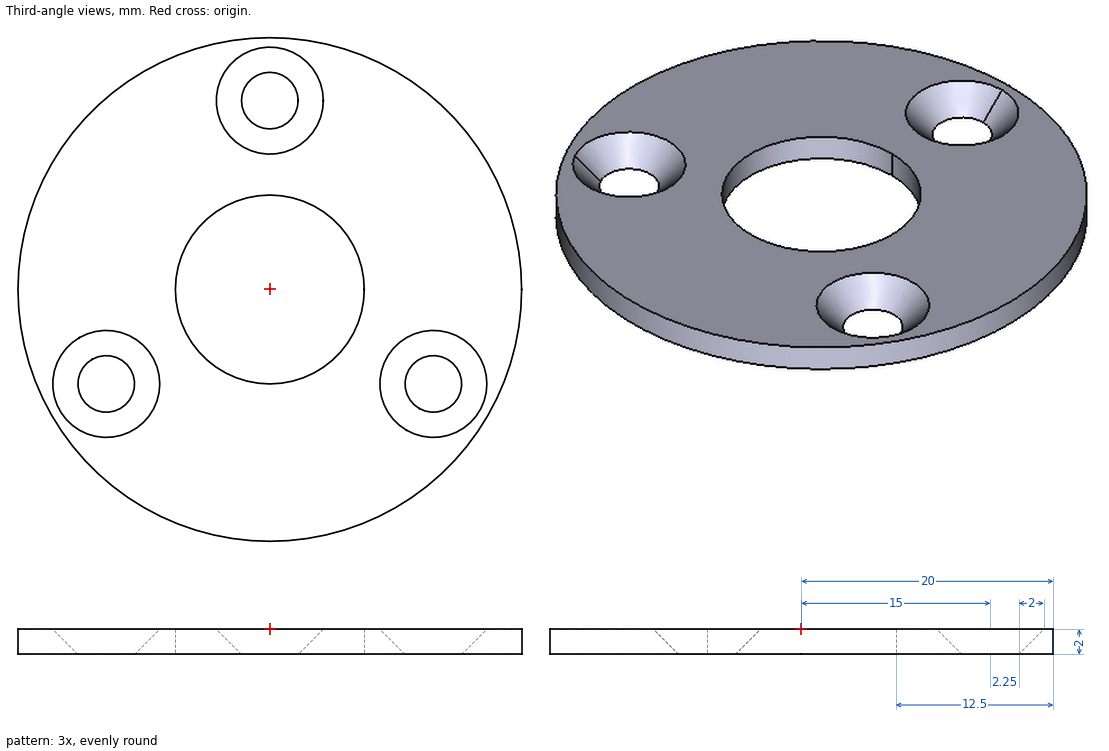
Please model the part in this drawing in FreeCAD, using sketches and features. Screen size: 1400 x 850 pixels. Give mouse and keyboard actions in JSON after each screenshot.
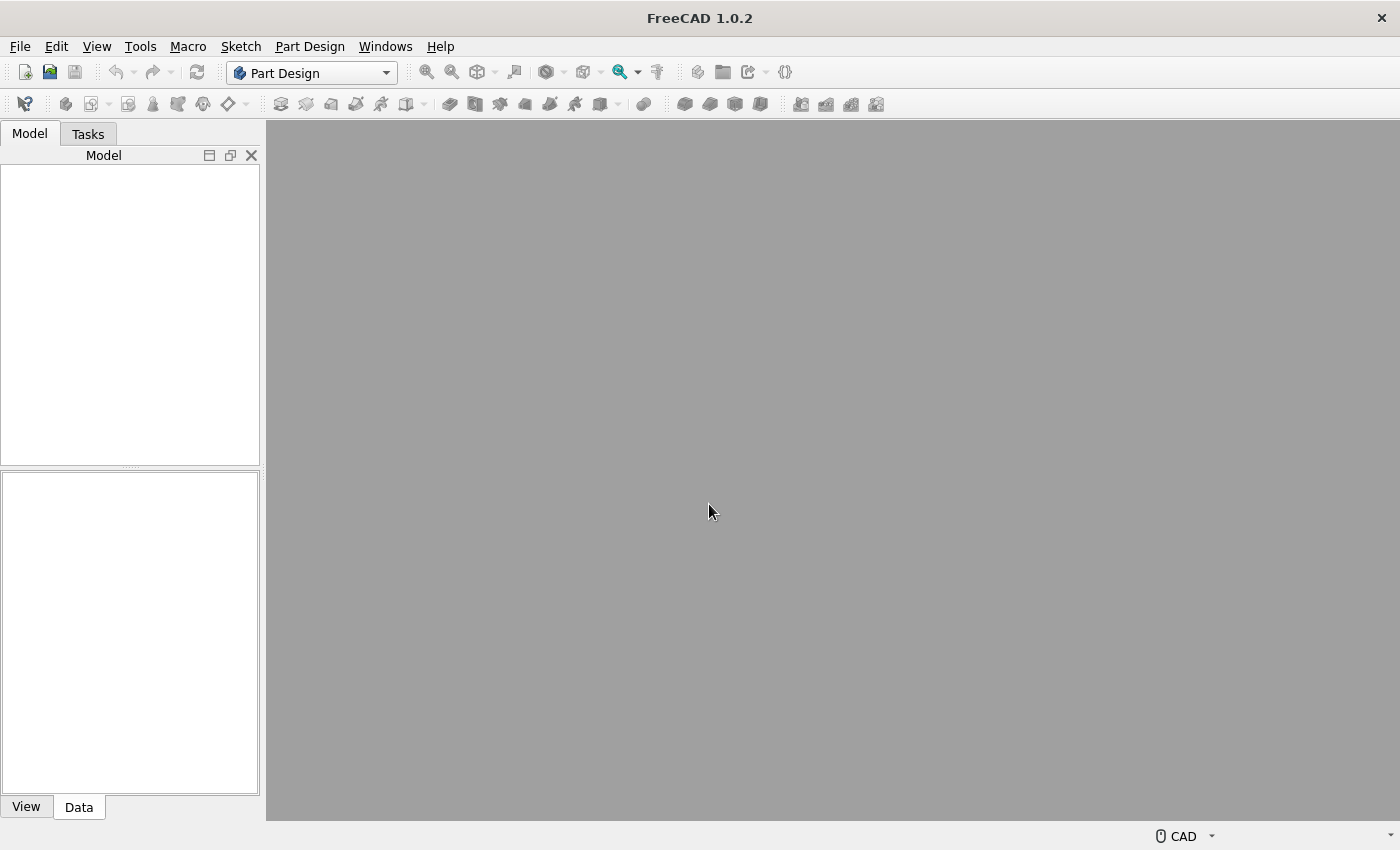
{"action": "left_click", "coordinate": [25, 72]}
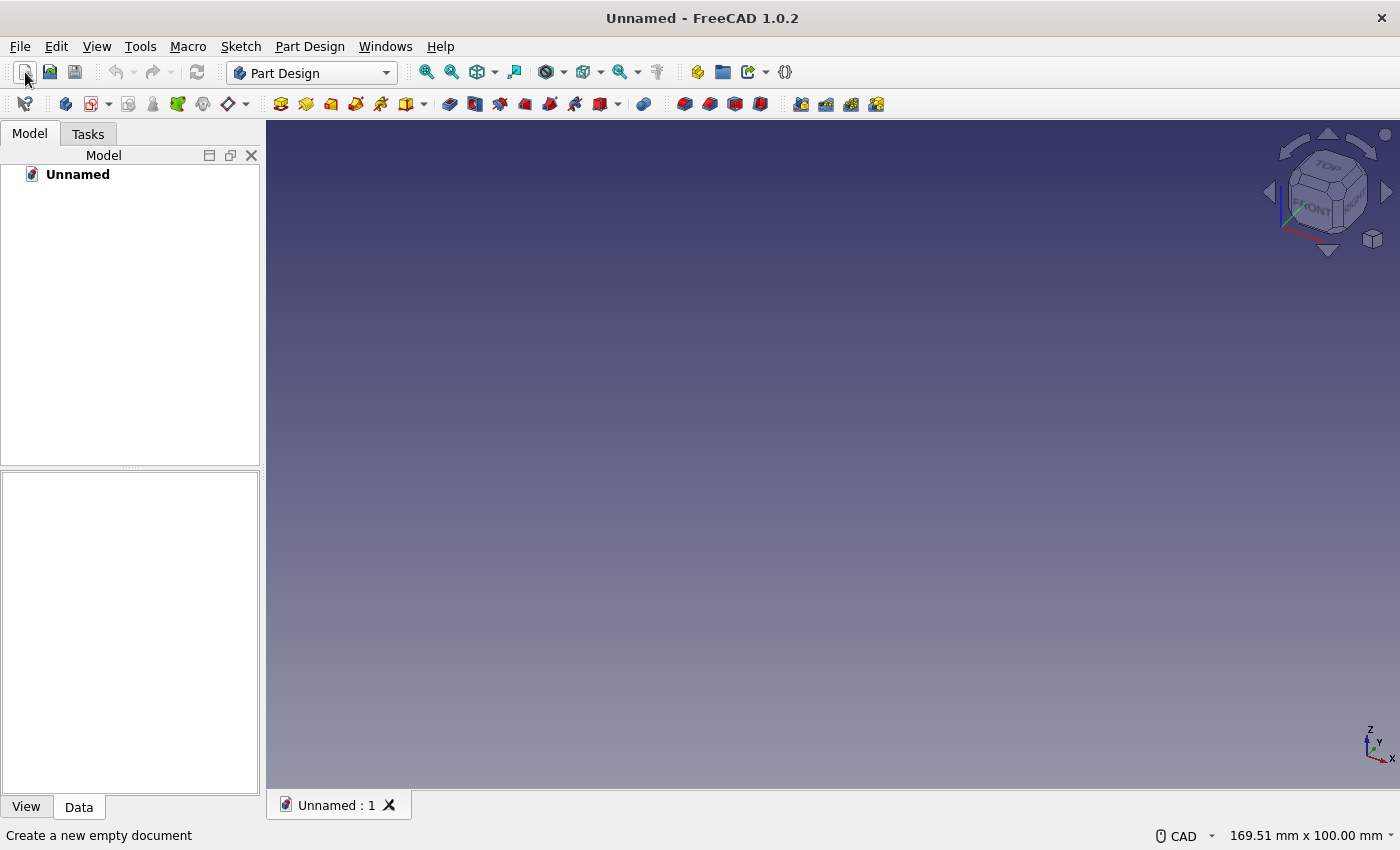
{"action": "left_click", "coordinate": [90, 104]}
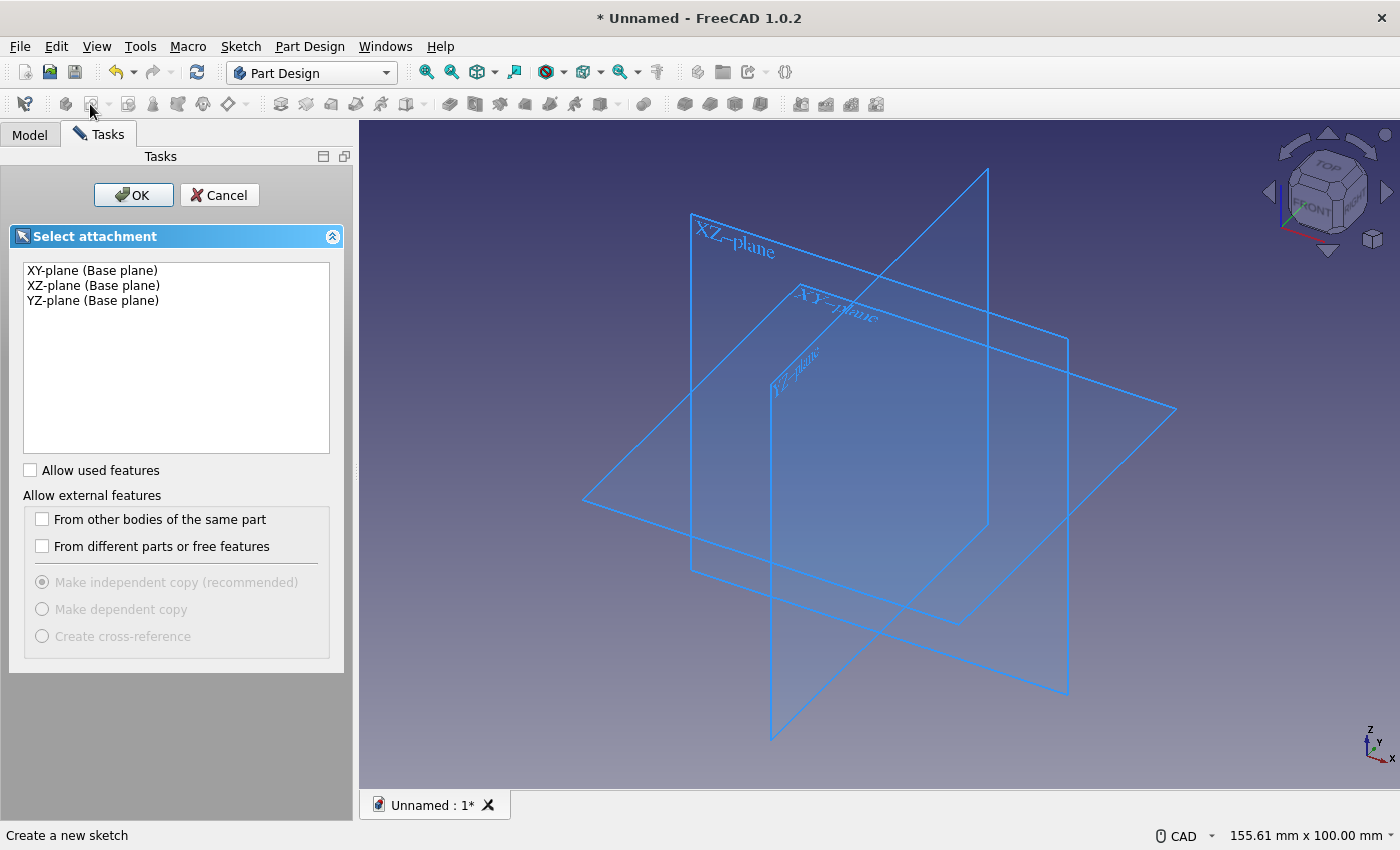
{"action": "left_click", "coordinate": [84, 300]}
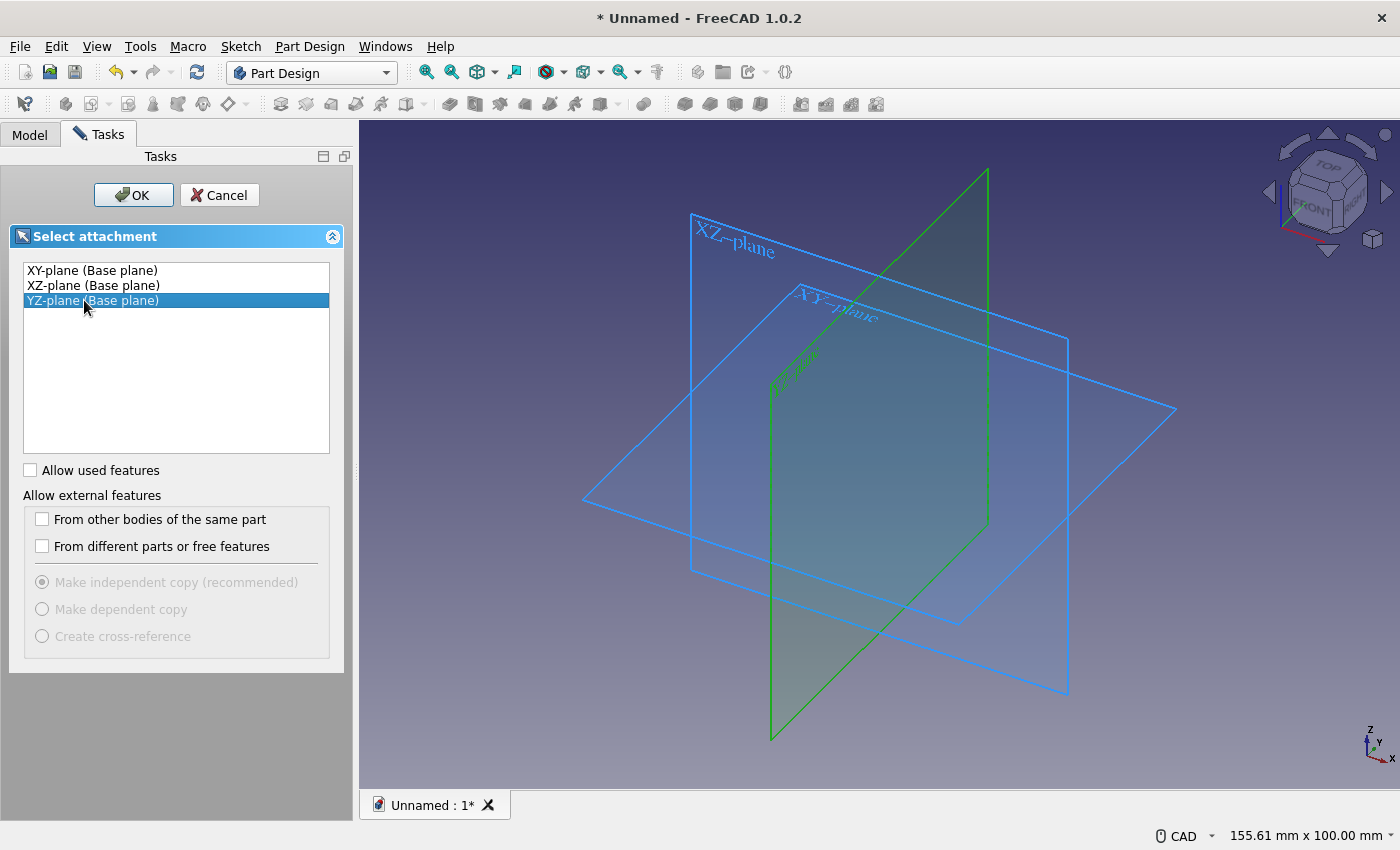
{"action": "left_click", "coordinate": [134, 195]}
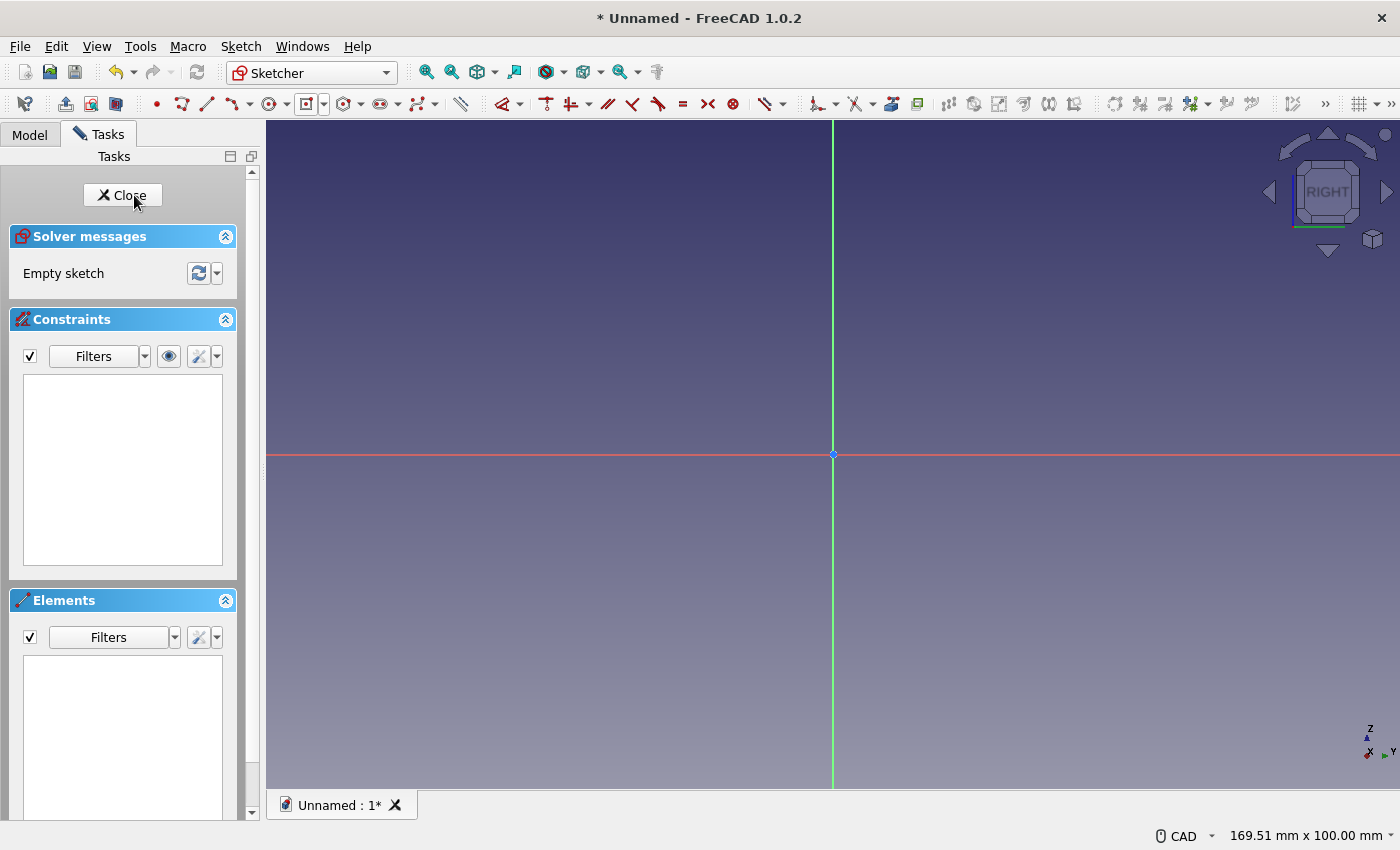
{"action": "scroll", "coordinate": [934, 463], "scroll_direction": "up", "scroll_amount": 8}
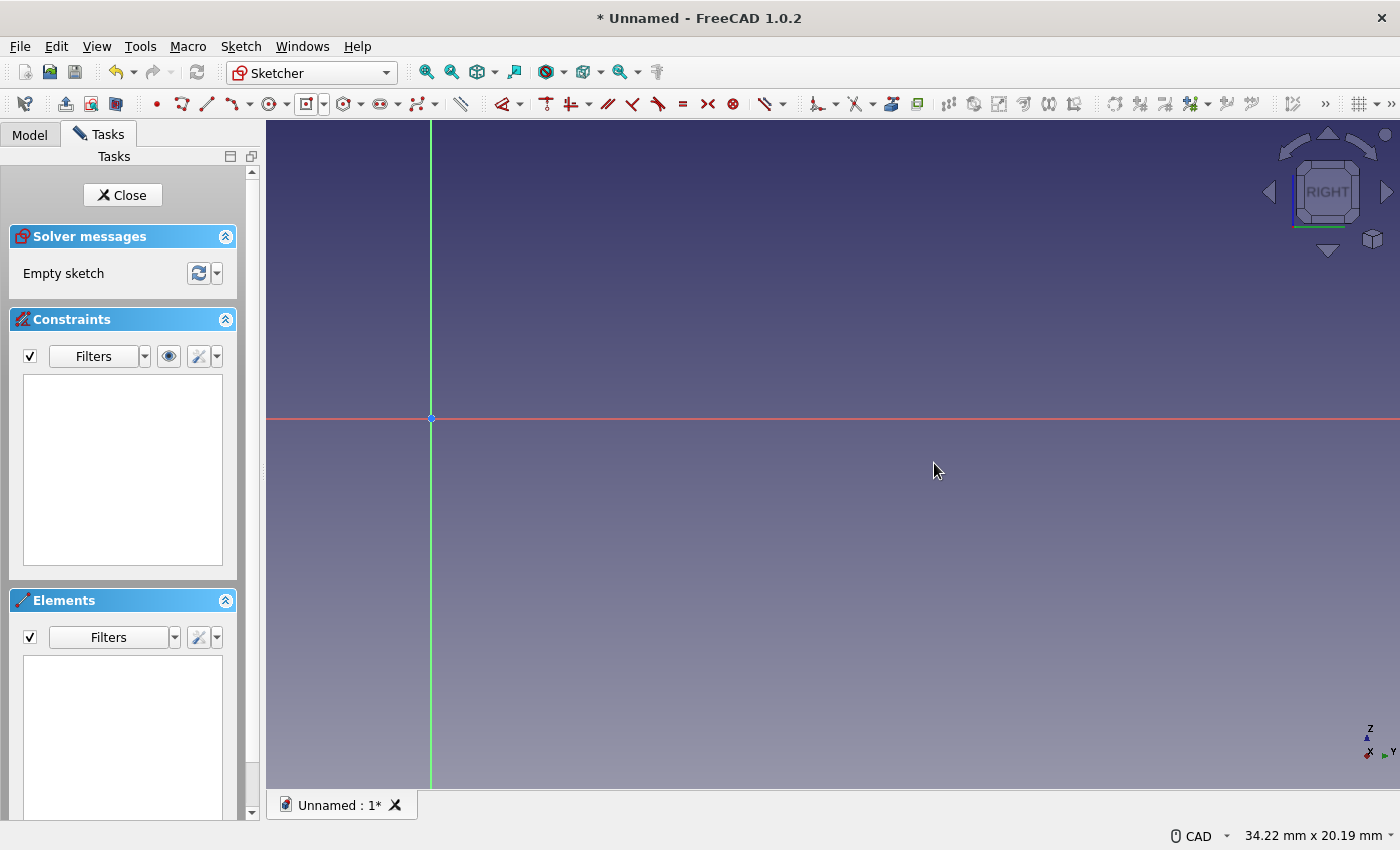
{"action": "key", "text": "g r"}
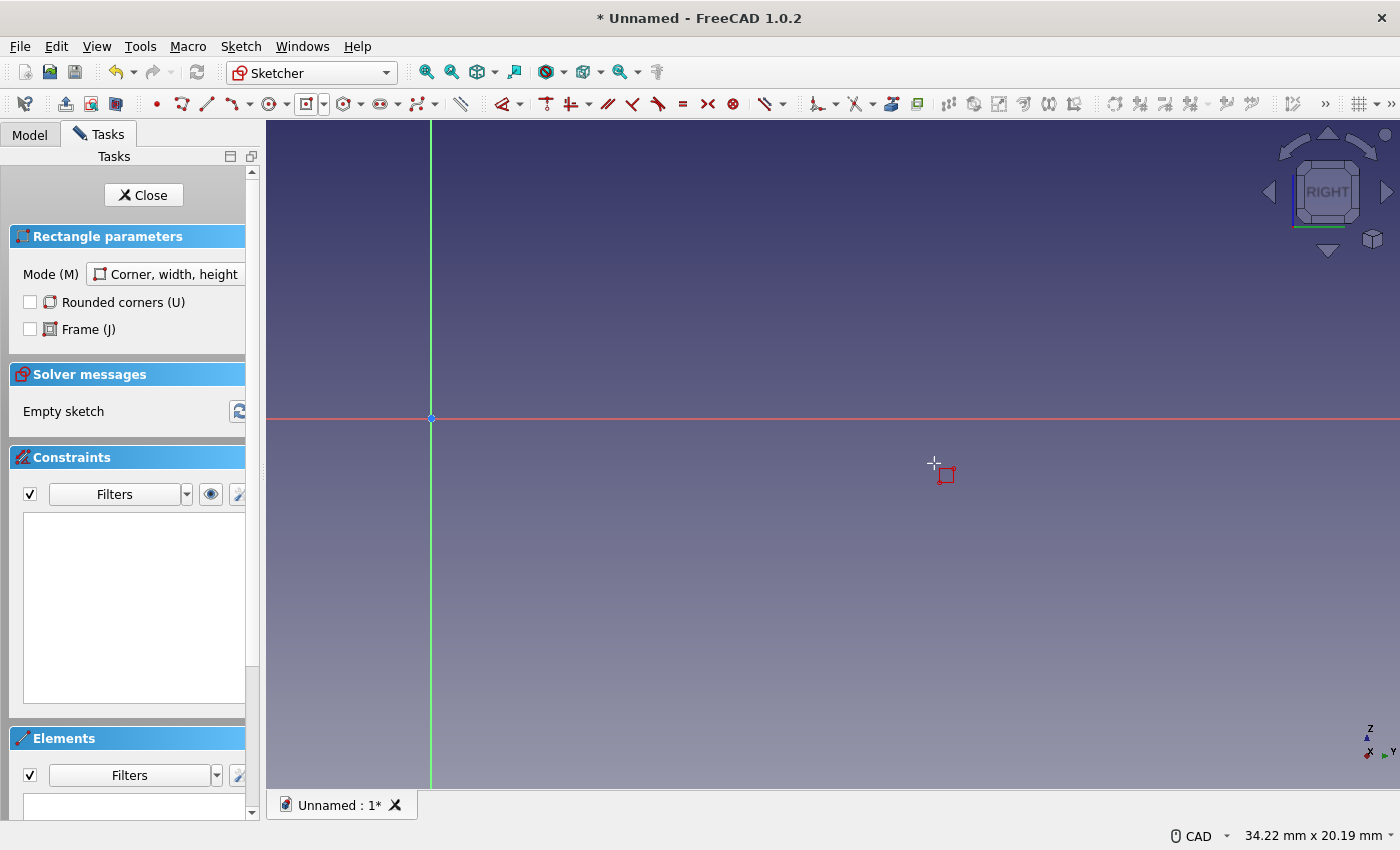
{"action": "left_click", "coordinate": [680, 419]}
{"action": "mouse_move", "coordinate": [1094, 485]}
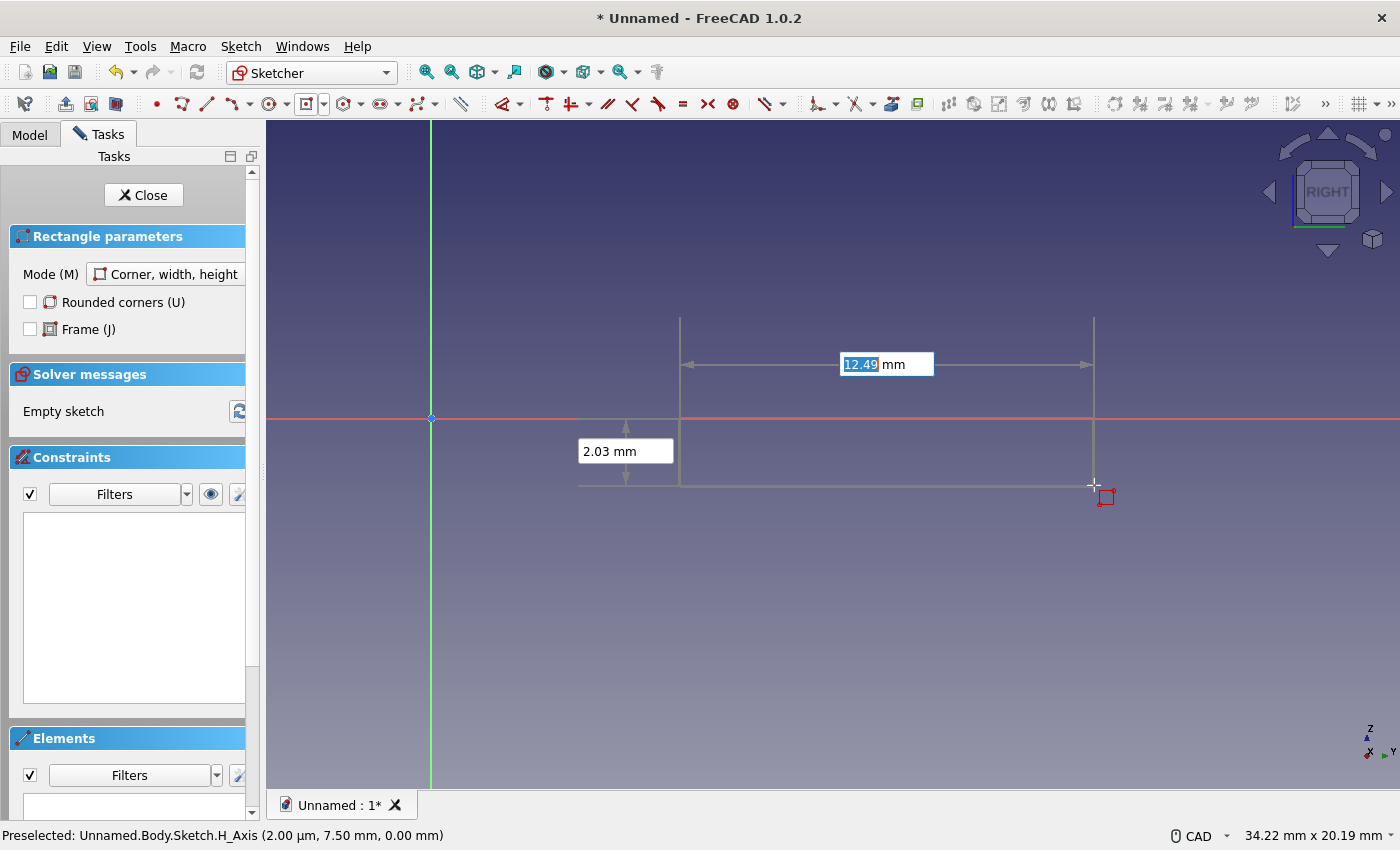
{"action": "type", "text": "12.5"}
{"action": "key", "text": "Tab"}
{"action": "type", "text": "2"}
{"action": "key", "text": "Return"}
{"action": "key", "text": "Escape"}